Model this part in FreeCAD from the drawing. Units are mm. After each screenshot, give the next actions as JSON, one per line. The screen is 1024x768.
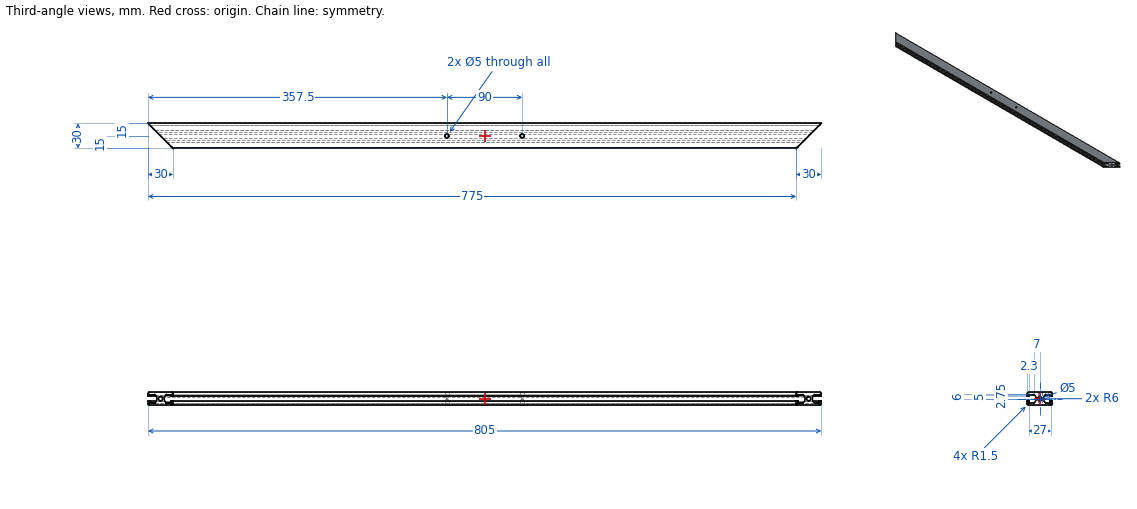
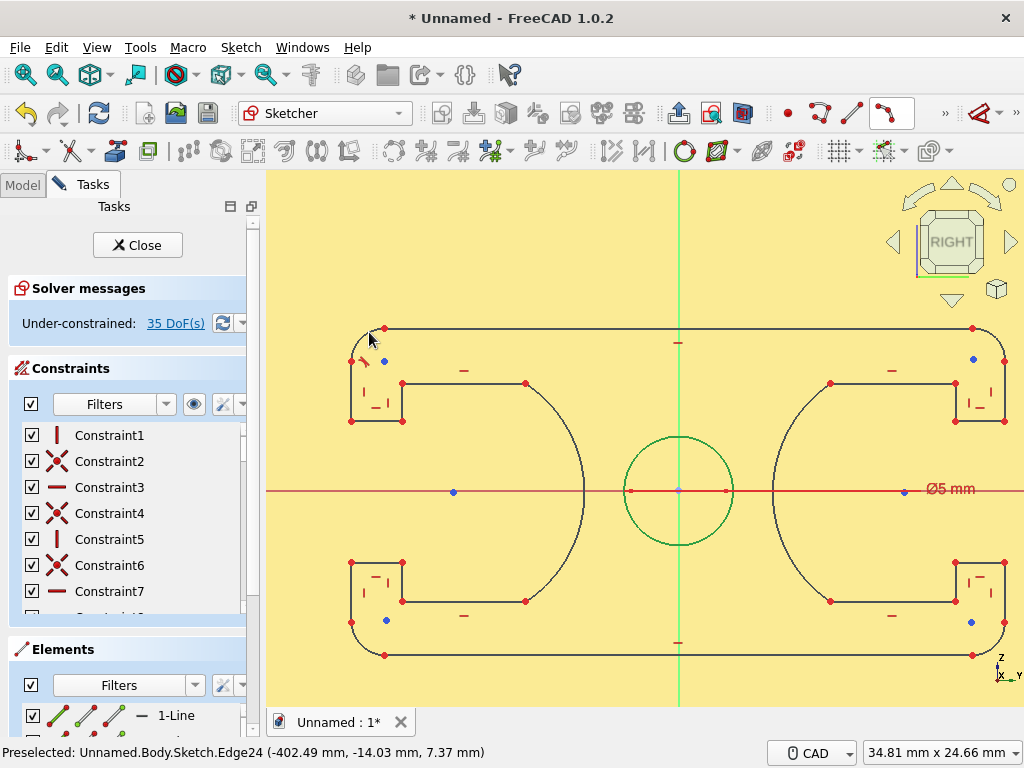
{"action": "left_click", "coordinate": [351, 581]}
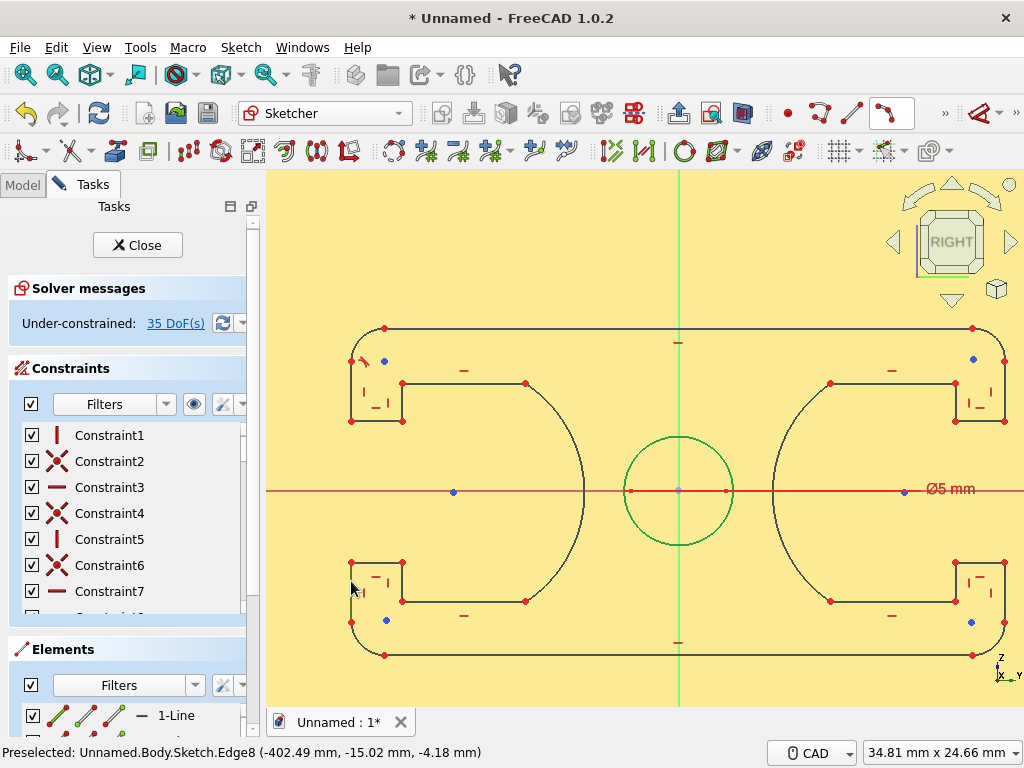
{"action": "left_click", "coordinate": [356, 637]}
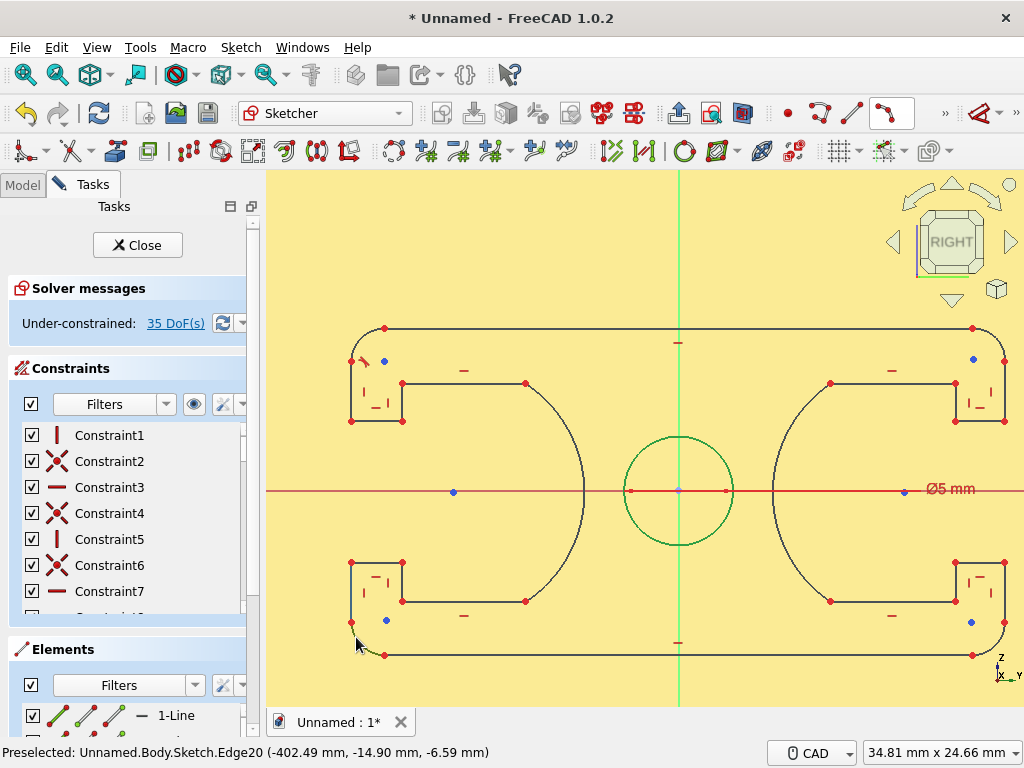
{"action": "key", "text": "t"}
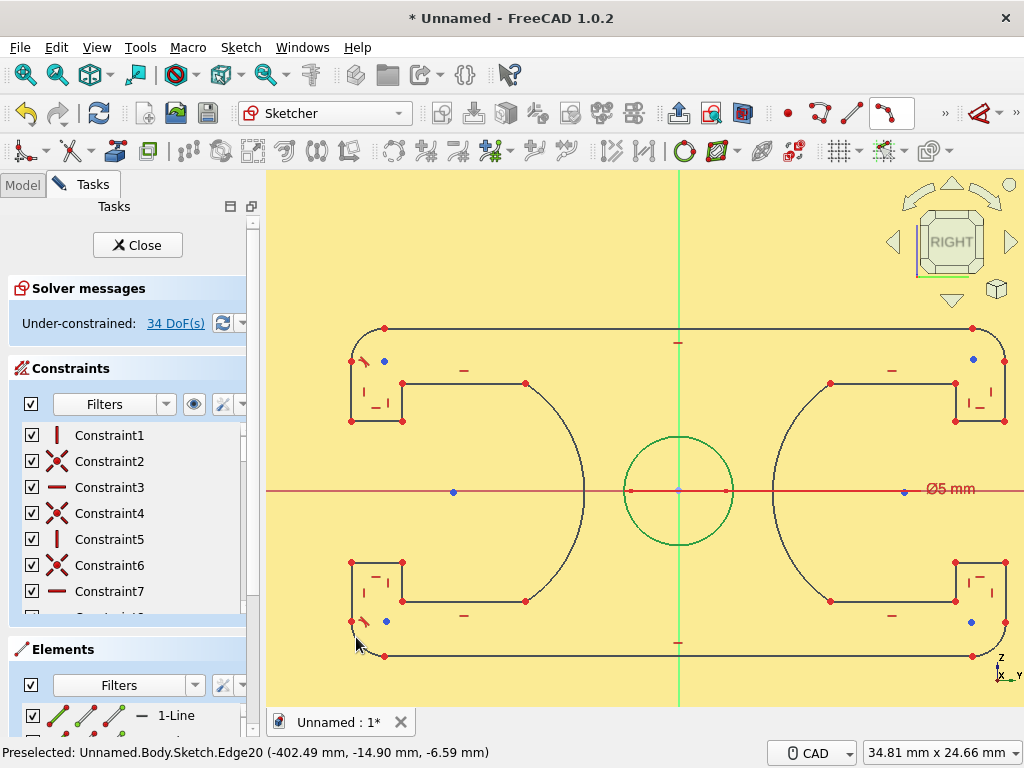
{"action": "left_click", "coordinate": [561, 656]}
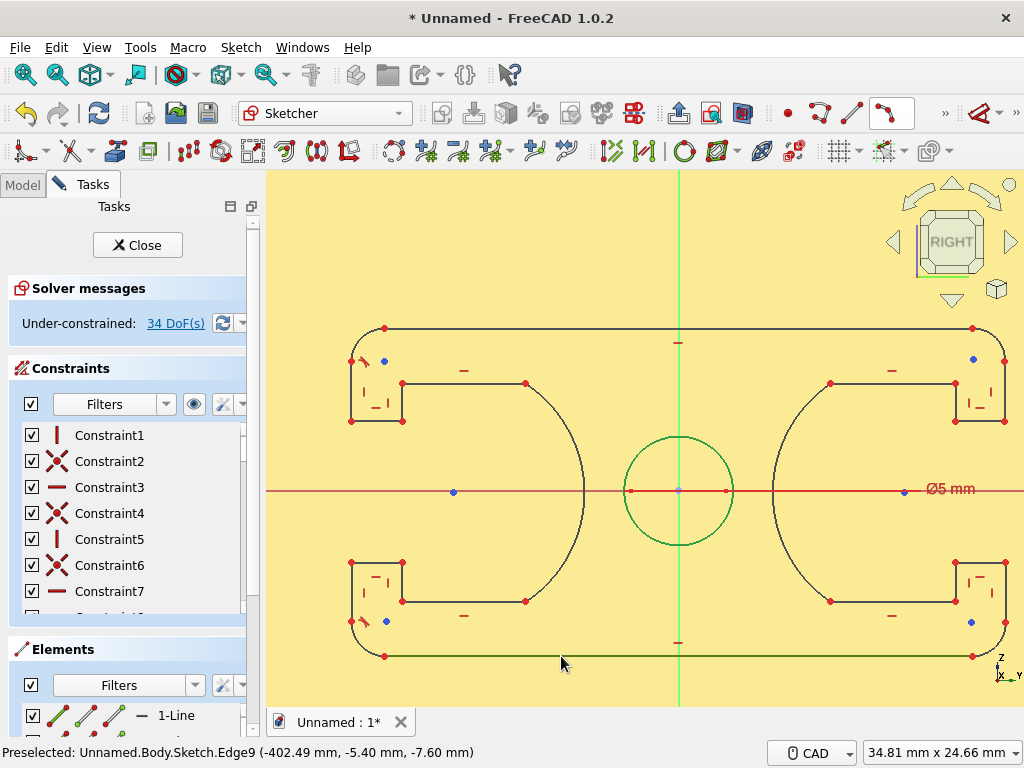
{"action": "left_click", "coordinate": [355, 637]}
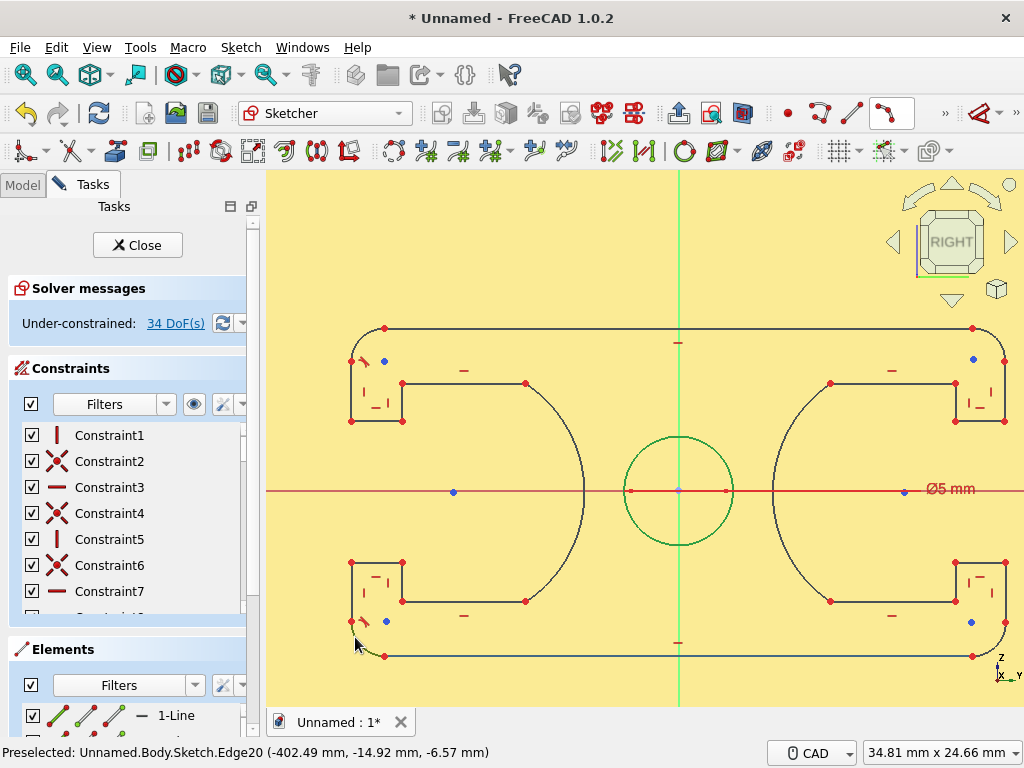
{"action": "key", "text": "t"}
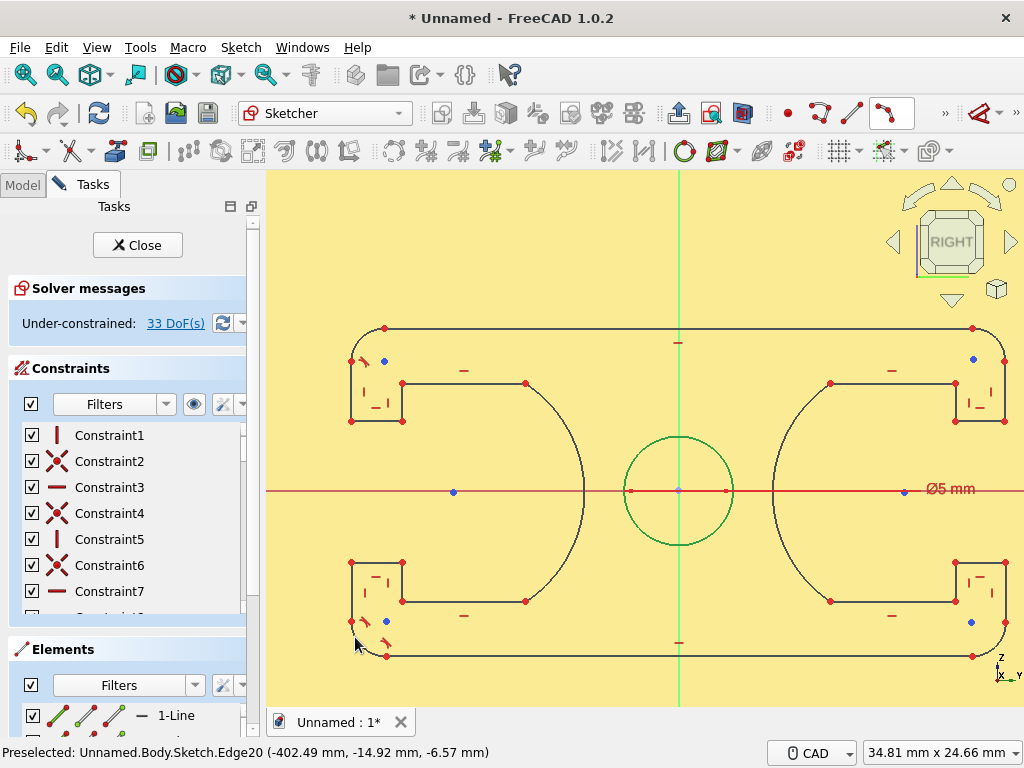
{"action": "left_click", "coordinate": [562, 656]}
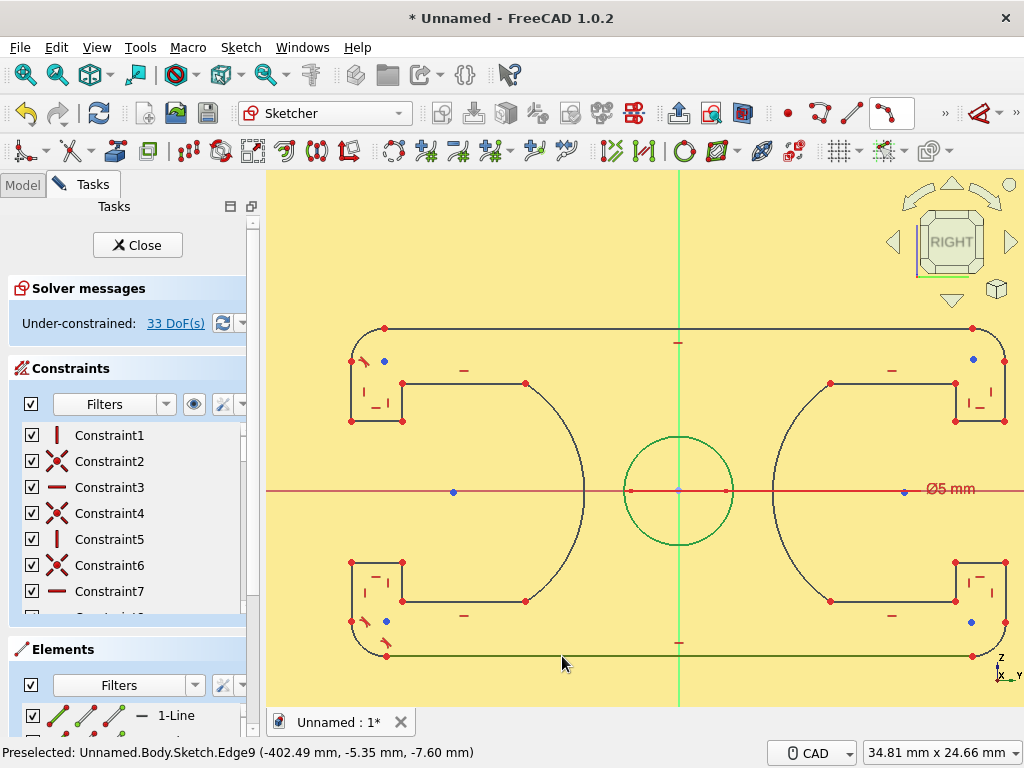
{"action": "scroll", "coordinate": [369, 332], "scroll_direction": "down", "scroll_amount": 2}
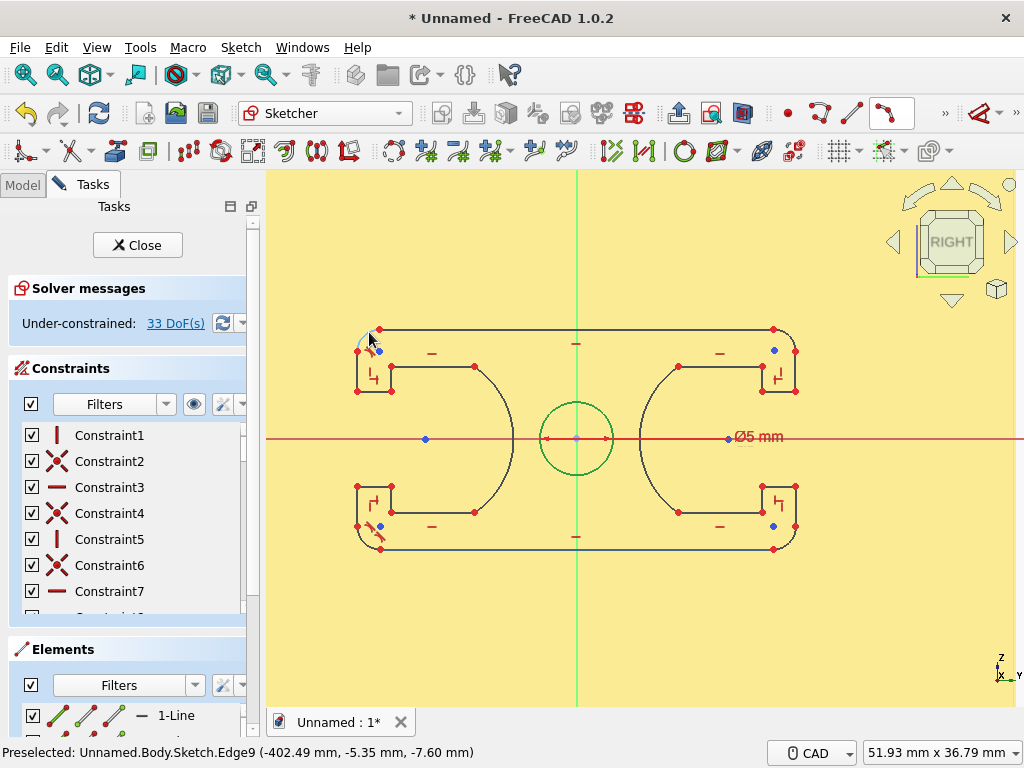
{"action": "scroll", "coordinate": [784, 547], "scroll_direction": "up", "scroll_amount": 2}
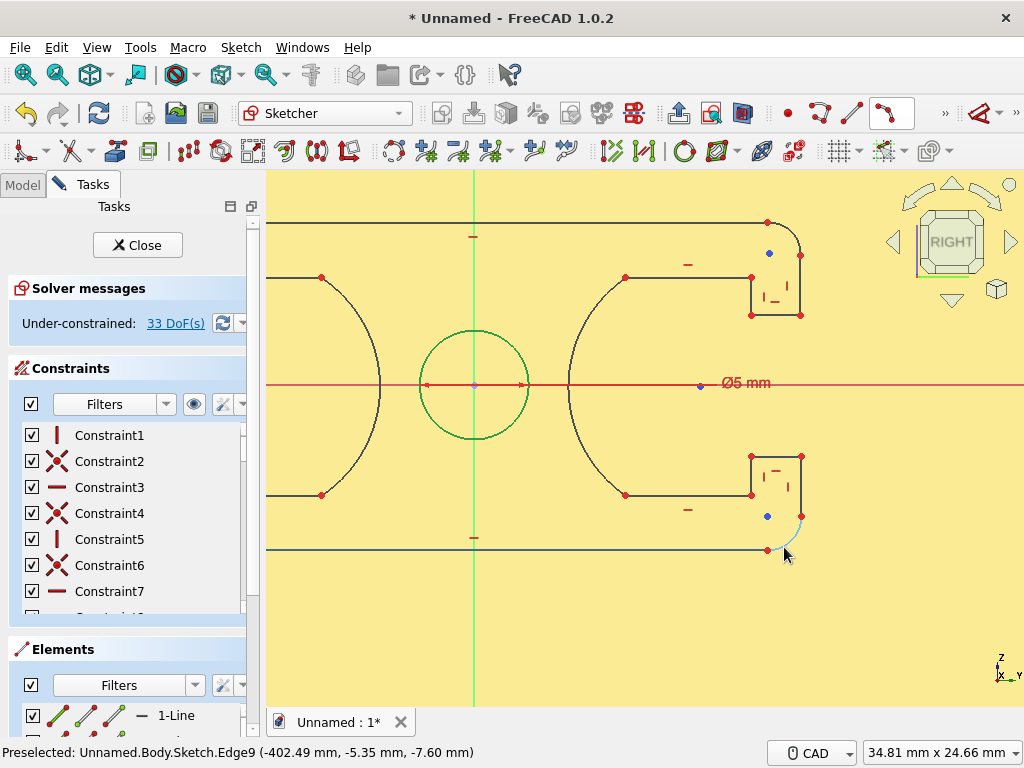
{"action": "left_click", "coordinate": [783, 547]}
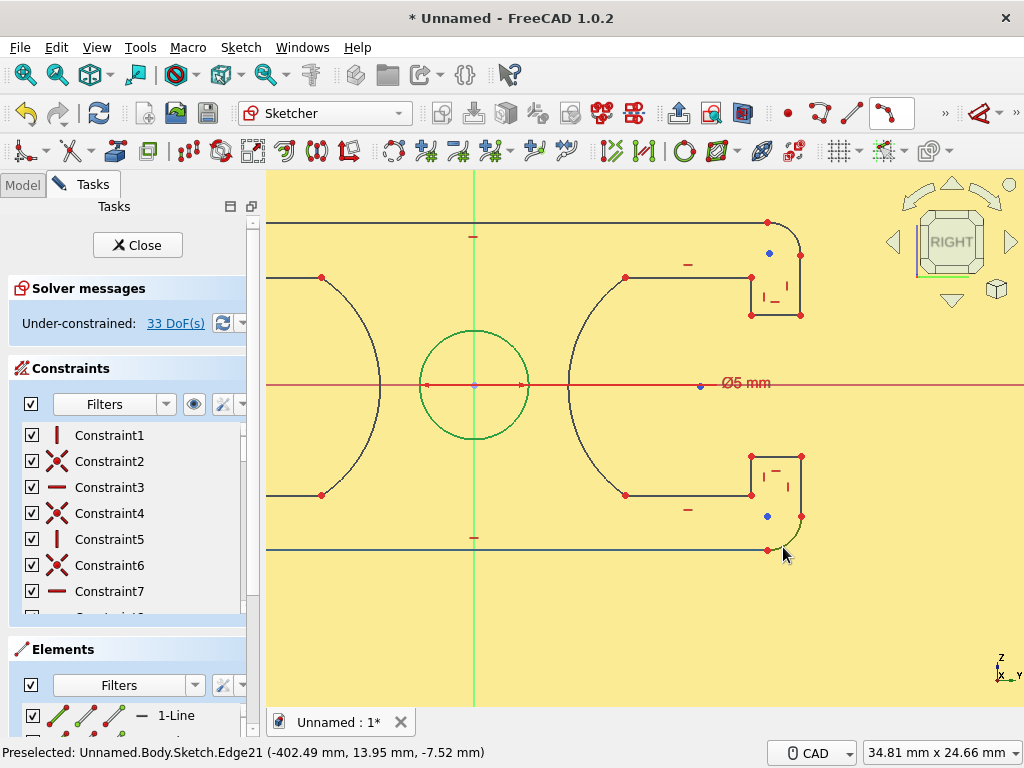
{"action": "key", "text": "t"}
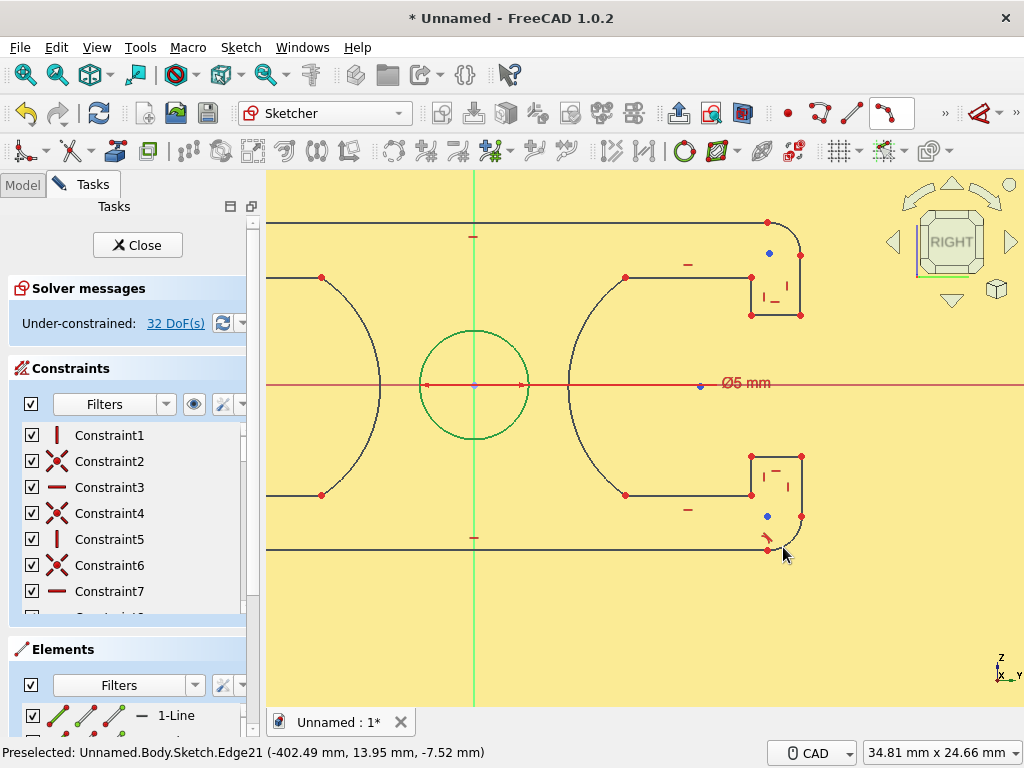
{"action": "left_click", "coordinate": [802, 499]}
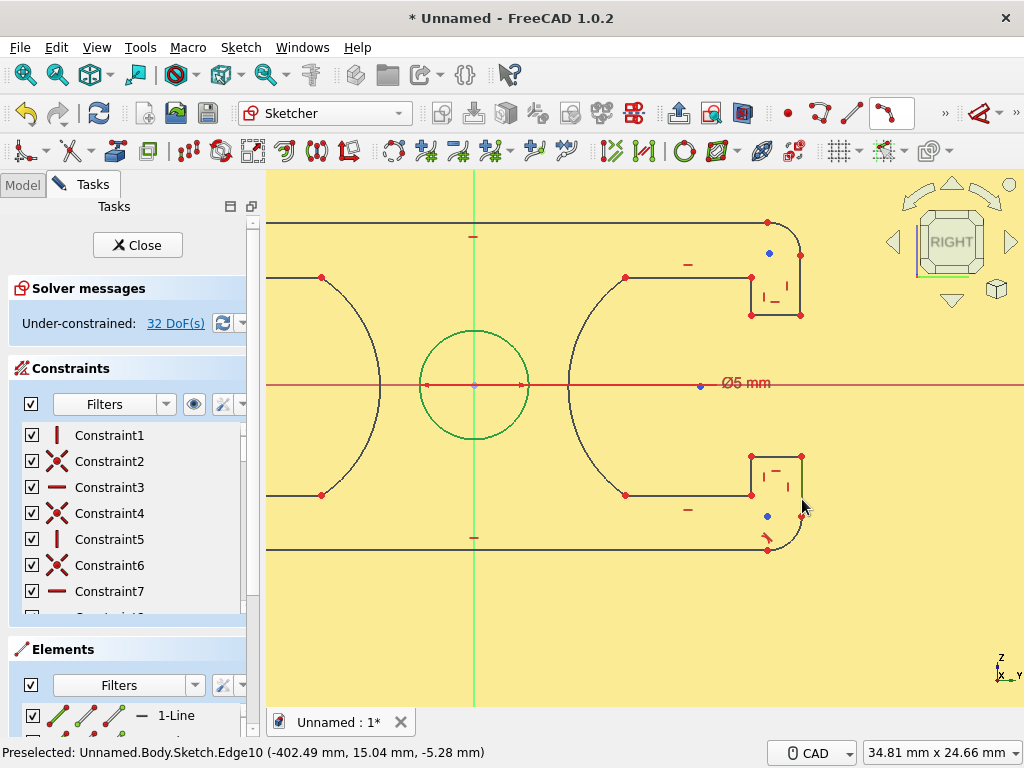
{"action": "left_click", "coordinate": [783, 547]}